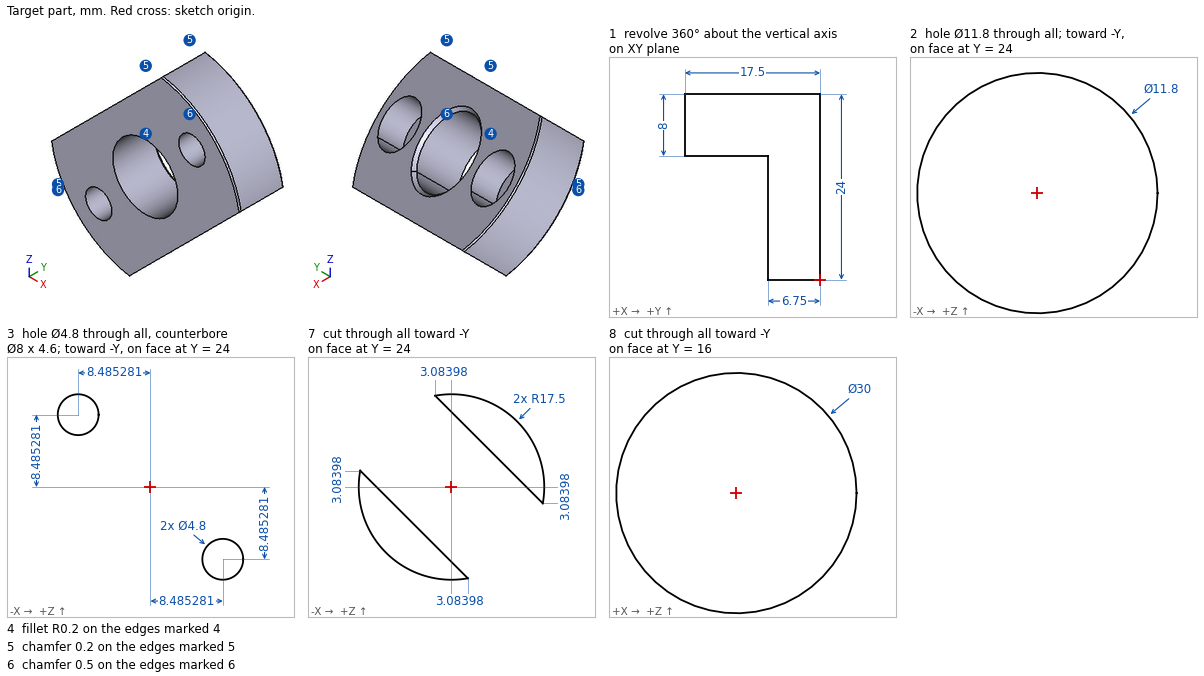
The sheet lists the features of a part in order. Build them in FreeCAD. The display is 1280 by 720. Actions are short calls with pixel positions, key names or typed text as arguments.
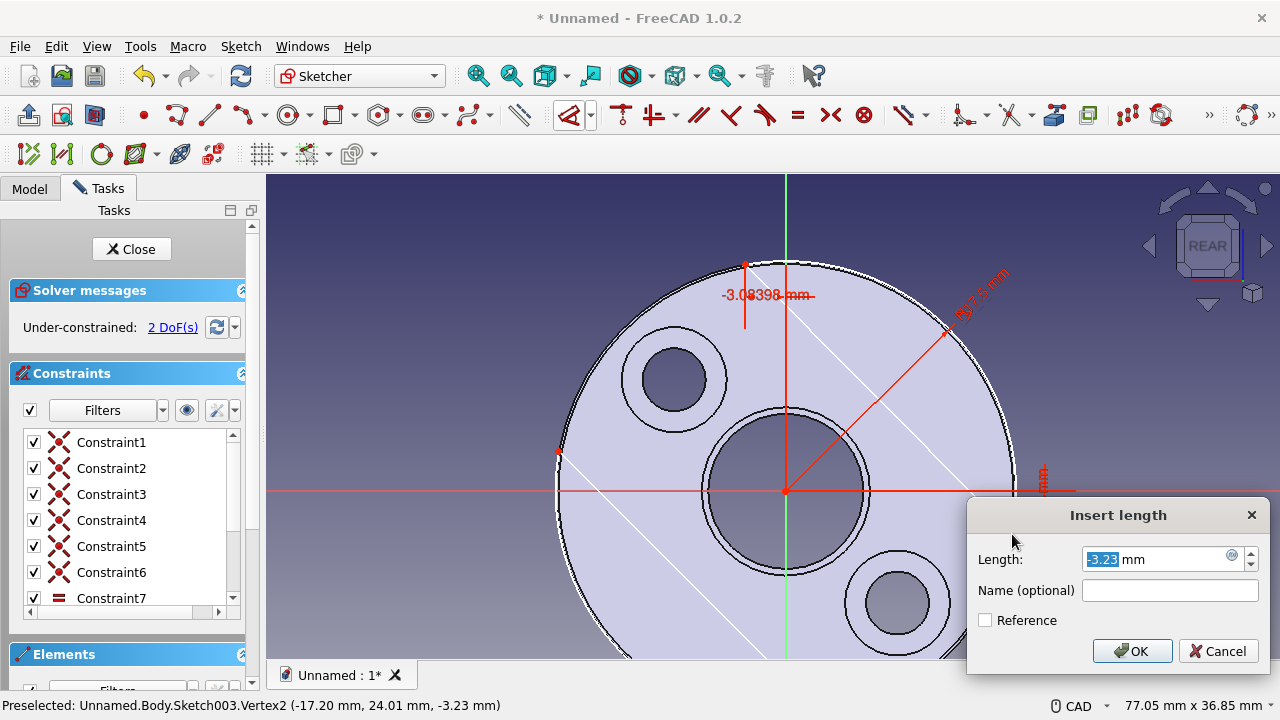
text(-3.08398)
key(Return)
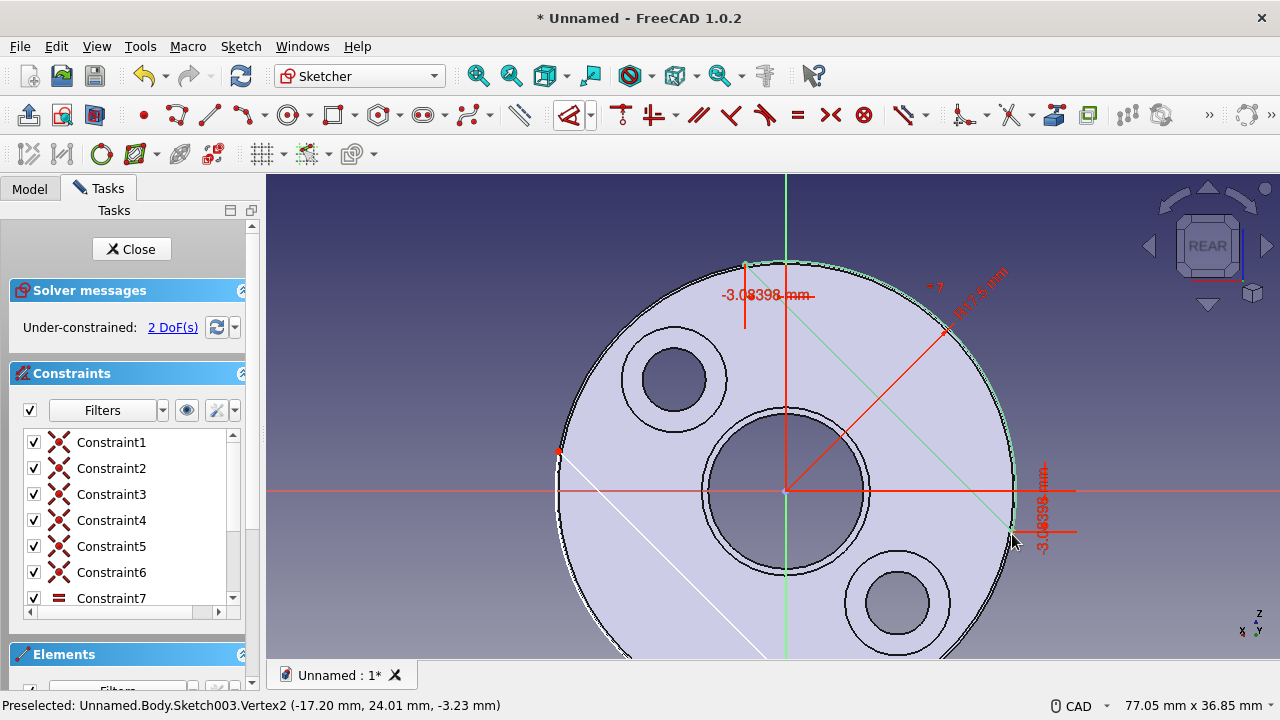
scroll(539, 264, down, 2)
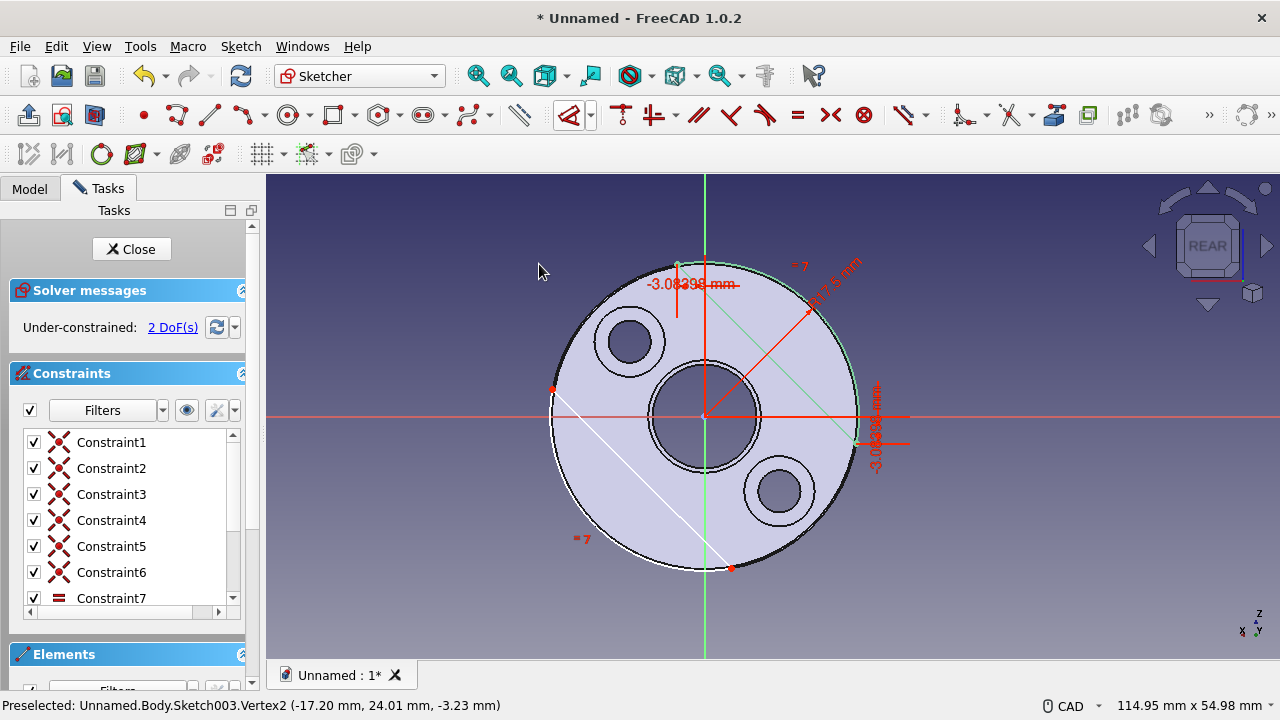
scroll(732, 568, up, 2)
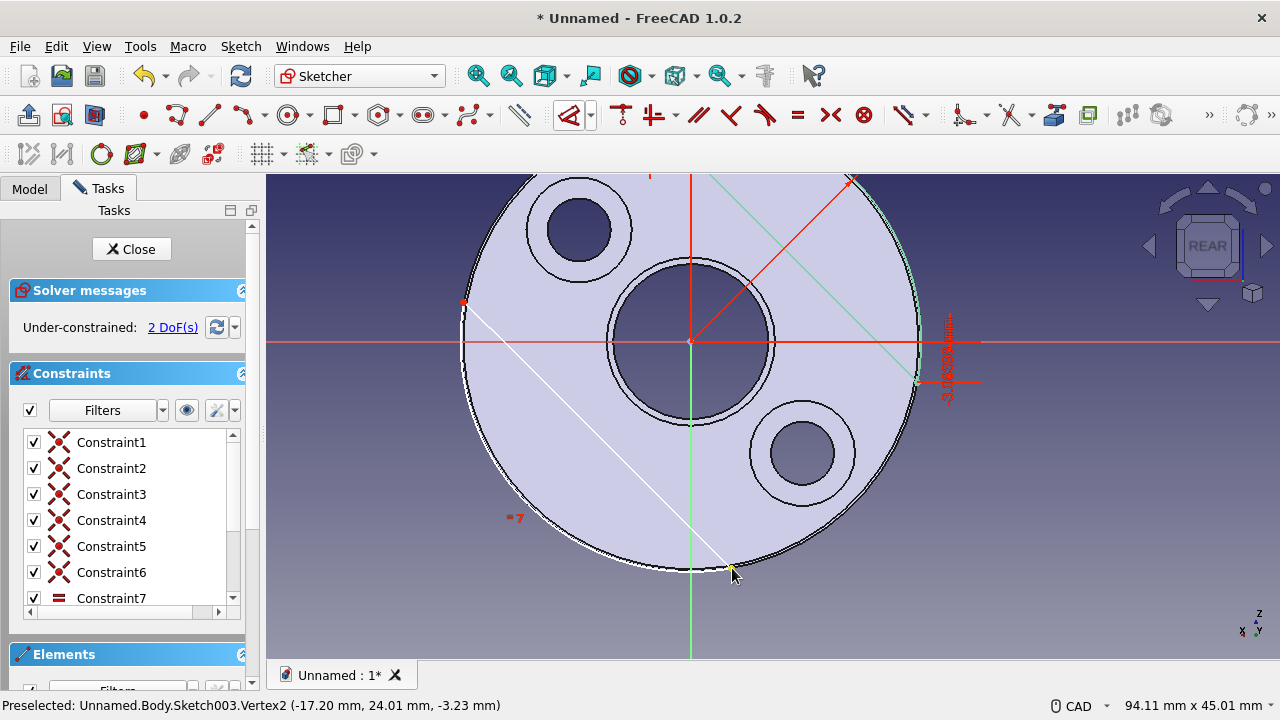
click(731, 568)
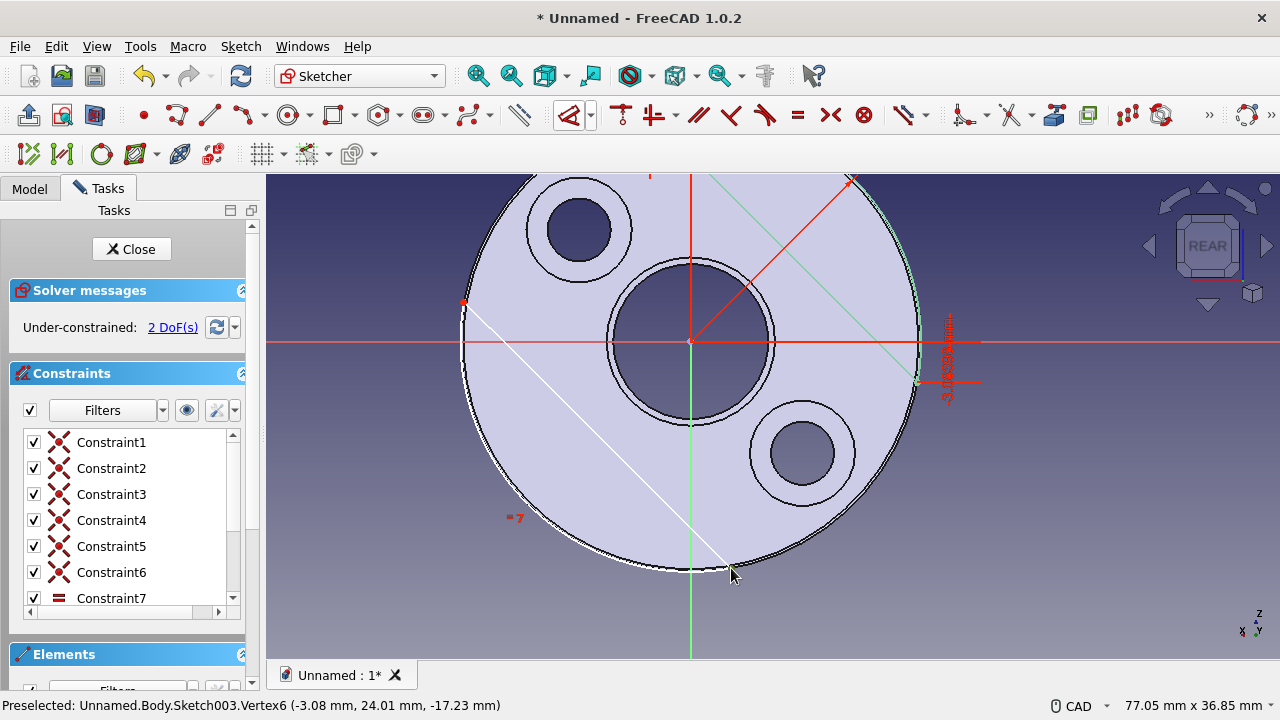
key(l)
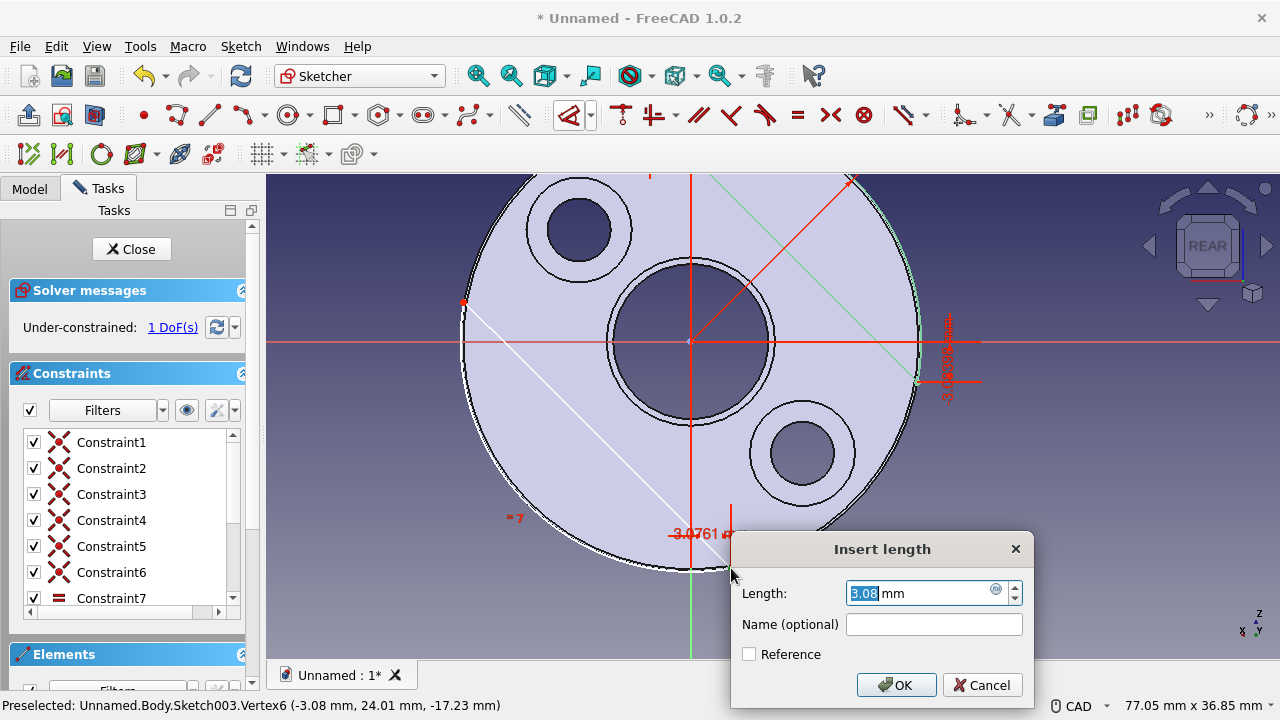
text(3.08398)
key(Return)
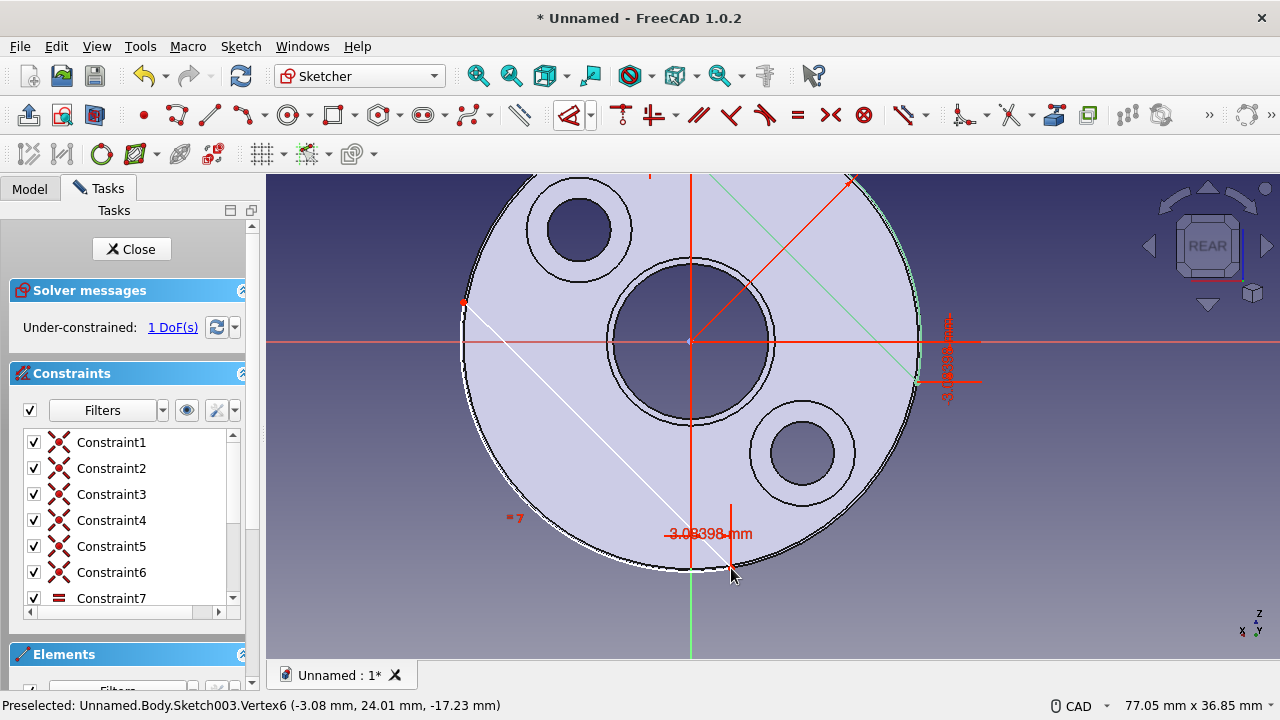
click(464, 302)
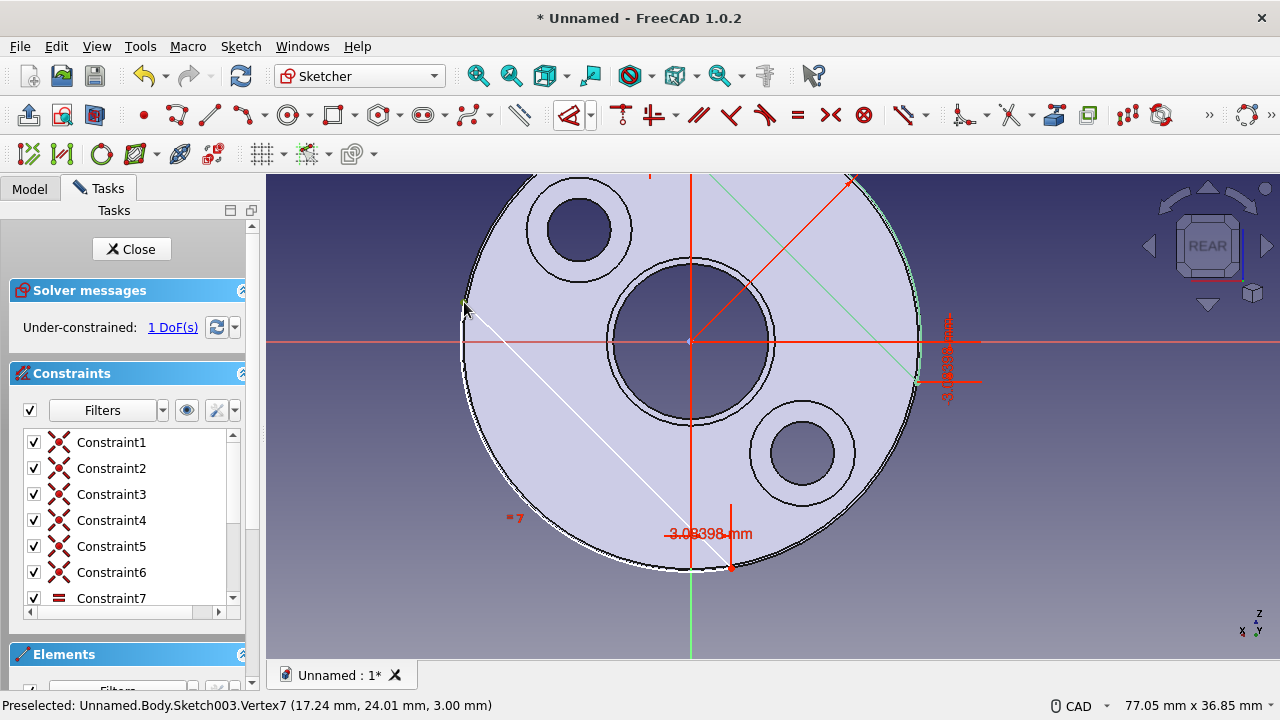
click(590, 116)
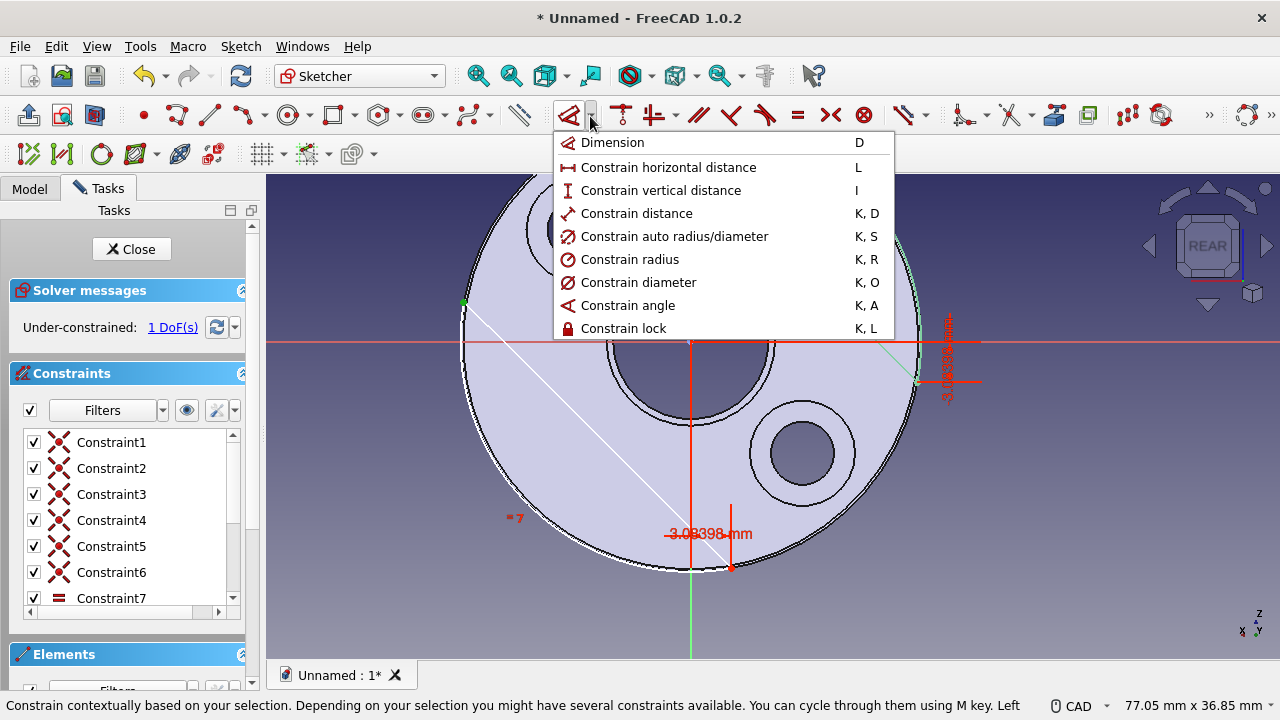
click(724, 190)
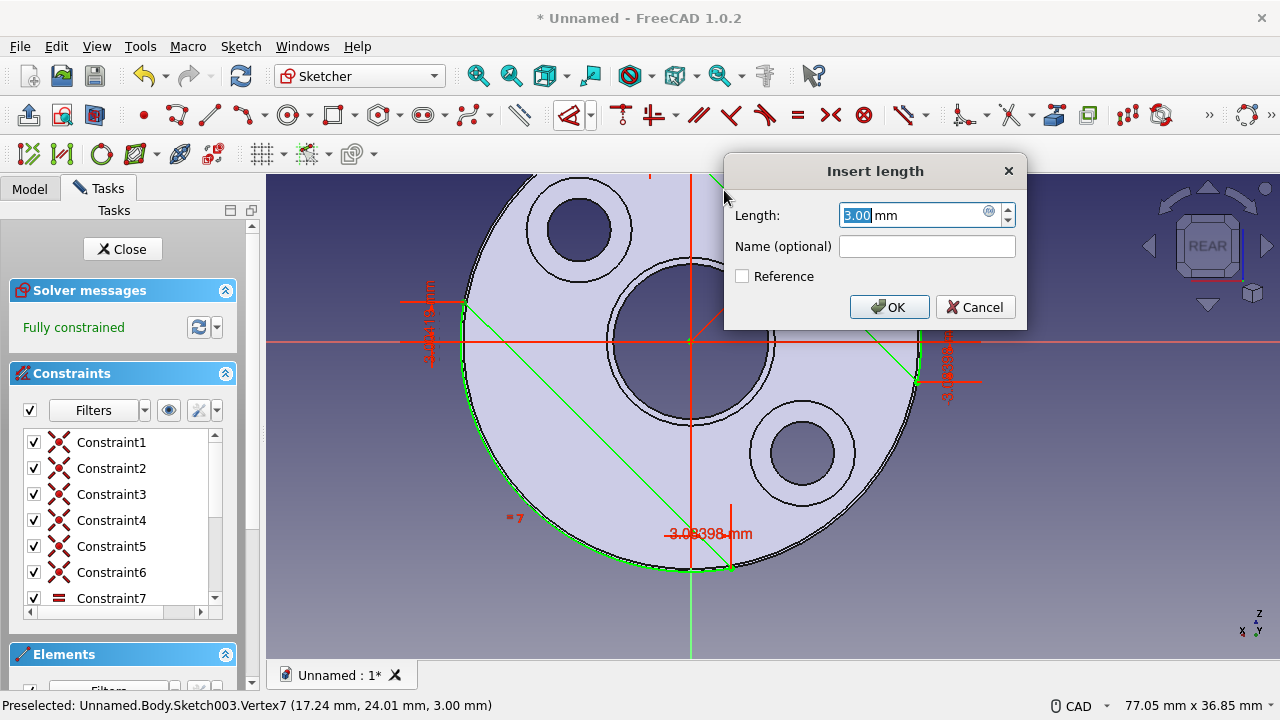
text(3.08398)
key(Return)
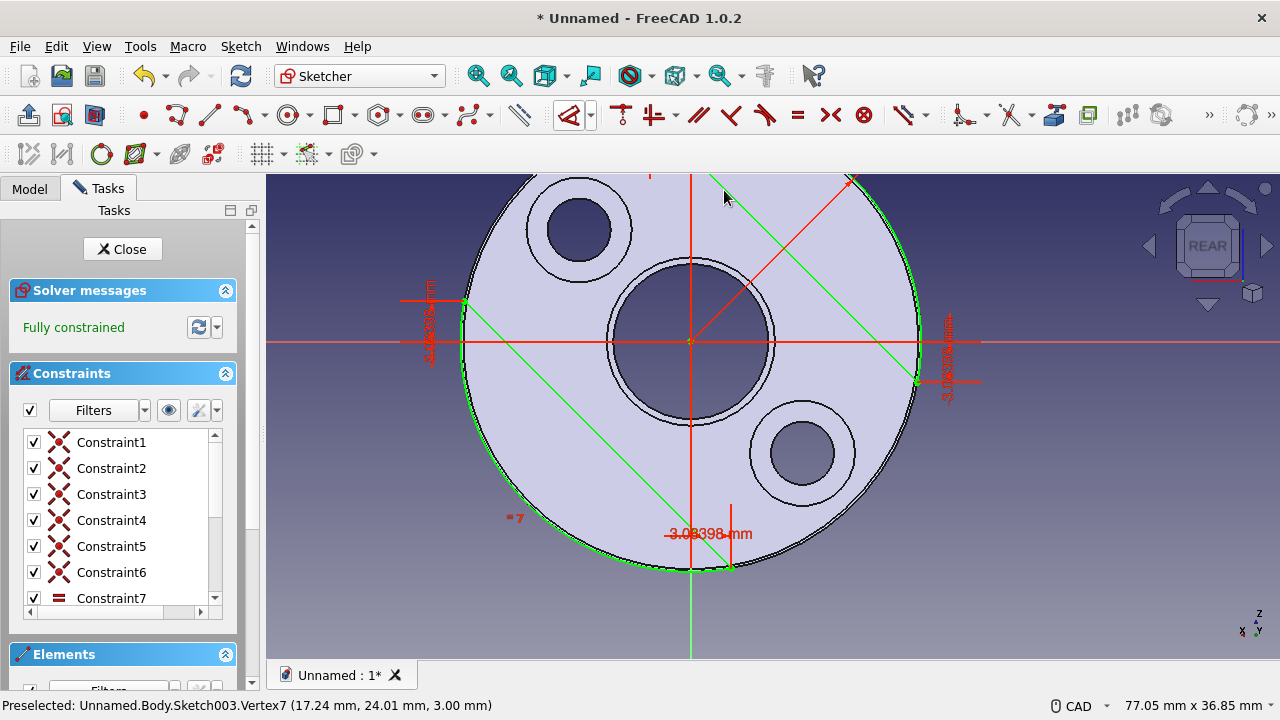
click(123, 249)